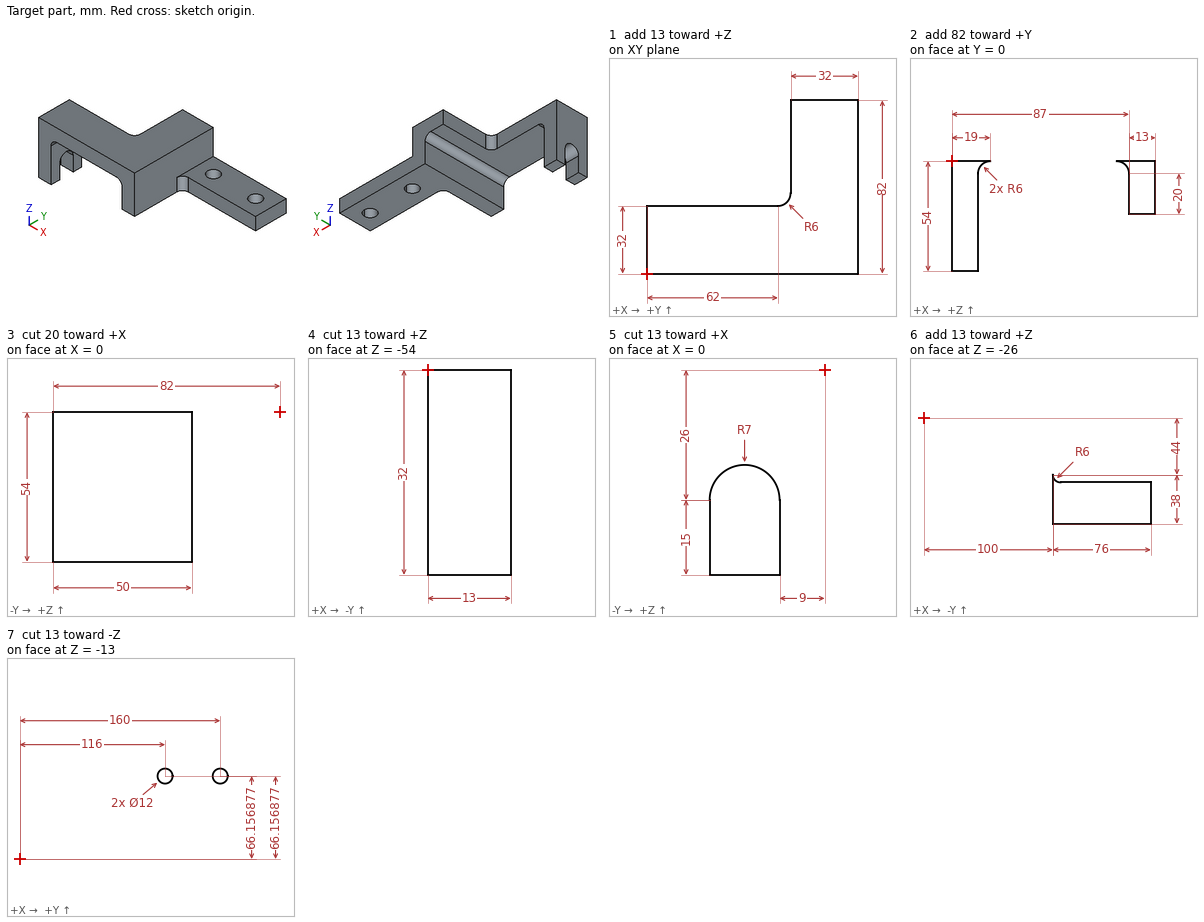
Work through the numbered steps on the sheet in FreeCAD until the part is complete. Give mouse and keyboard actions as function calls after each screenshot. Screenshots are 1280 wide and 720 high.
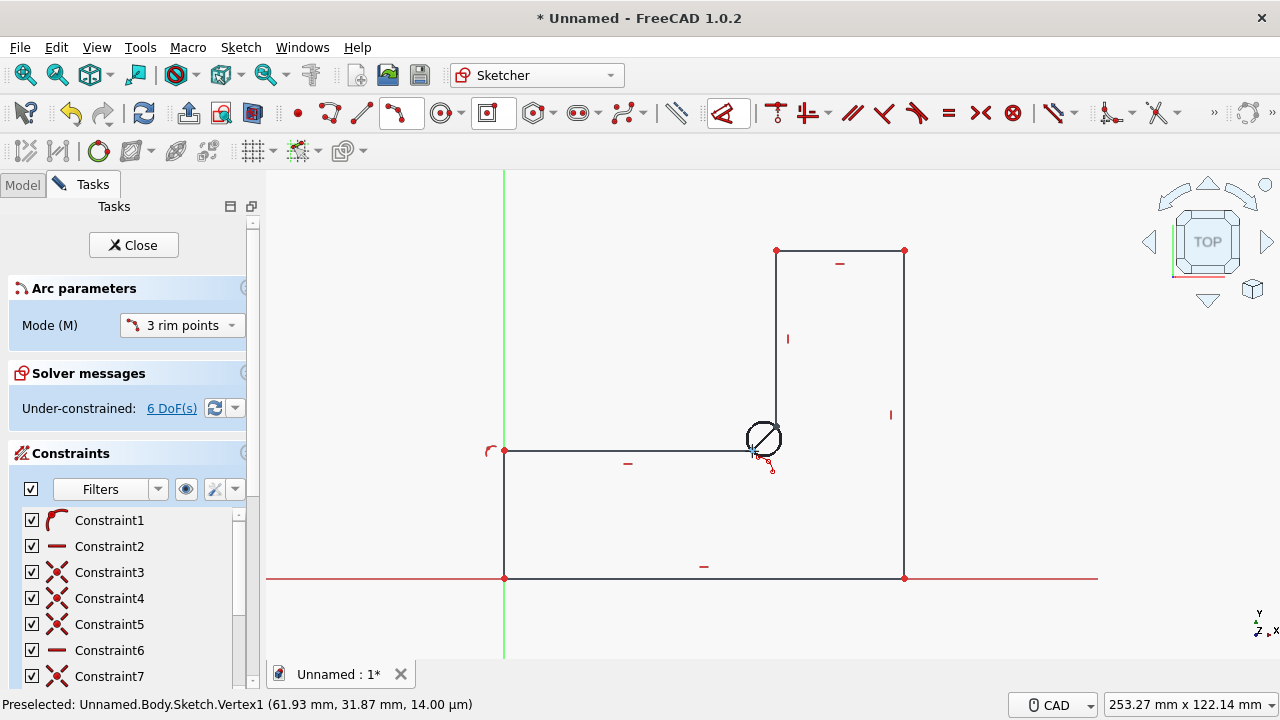
scroll(769, 443, up, 5)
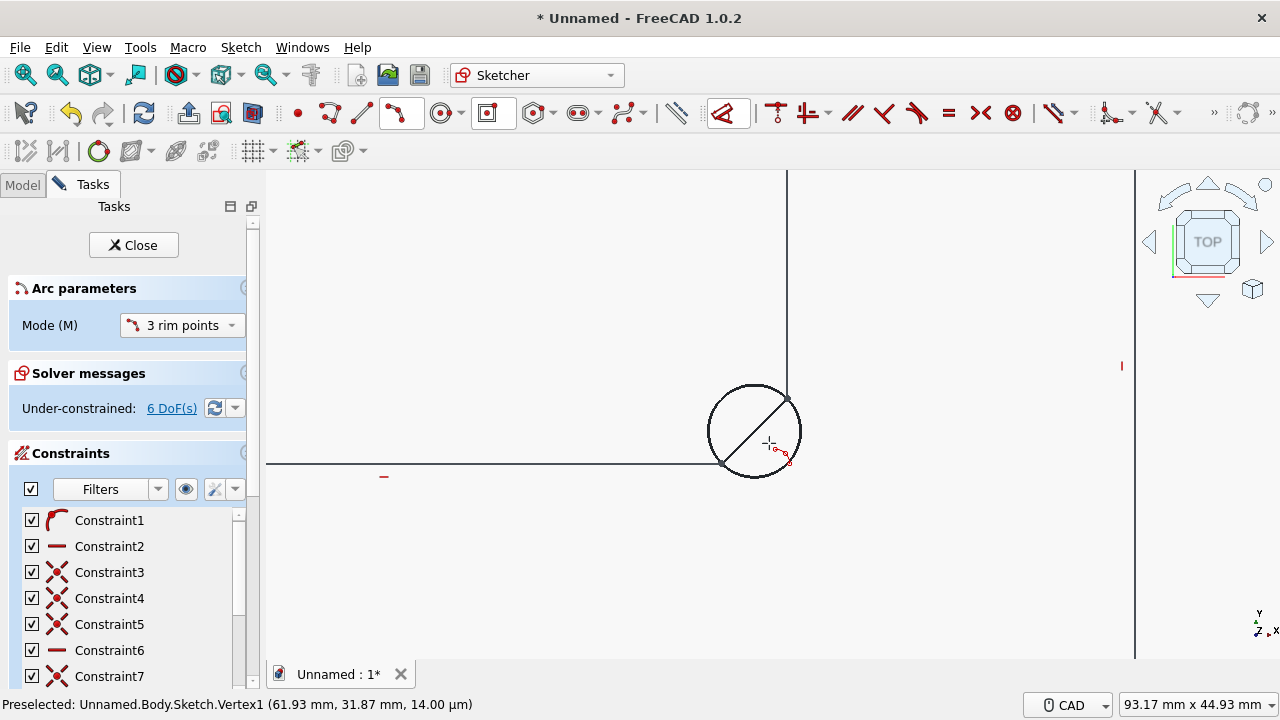
click(769, 443)
key(Escape)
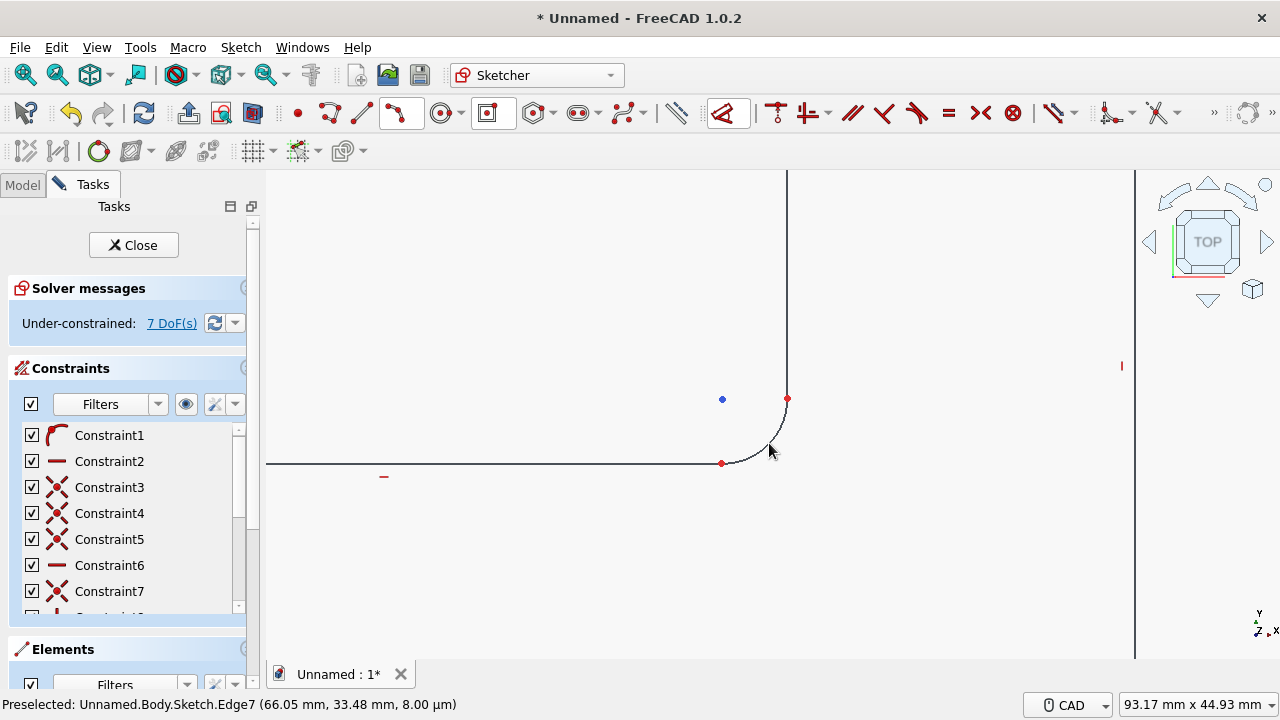
click(520, 464)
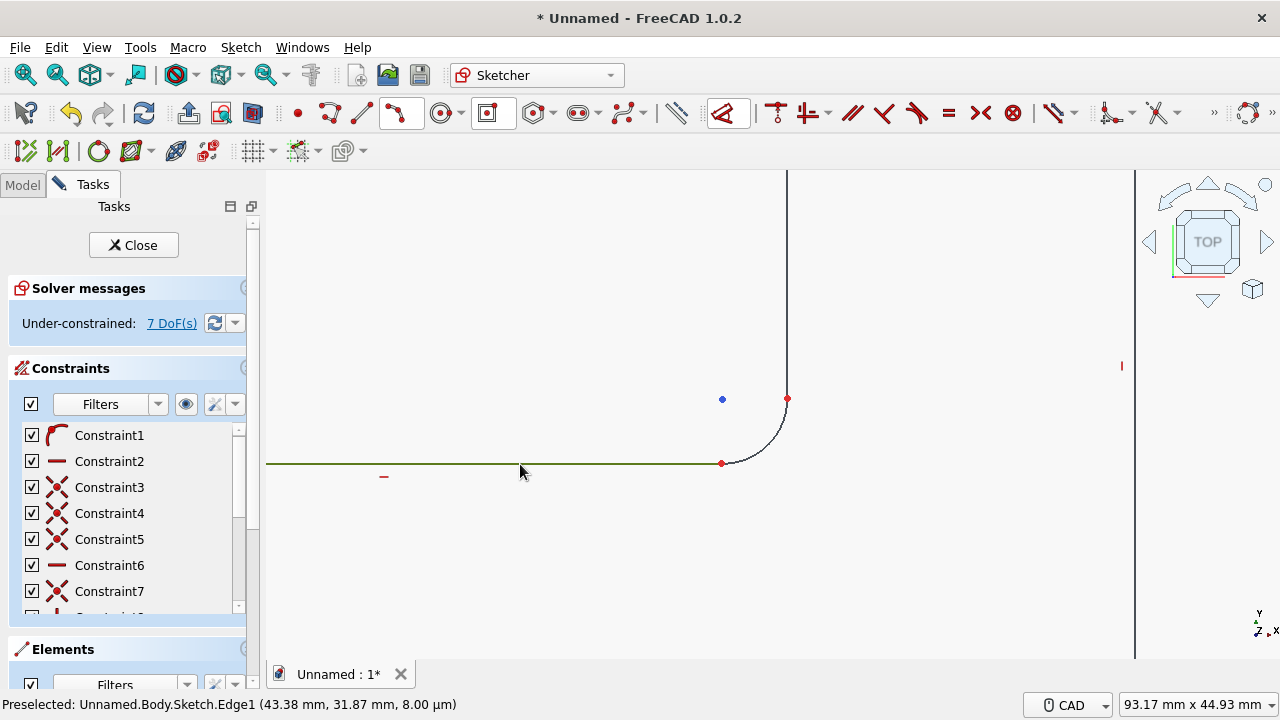
click(752, 457)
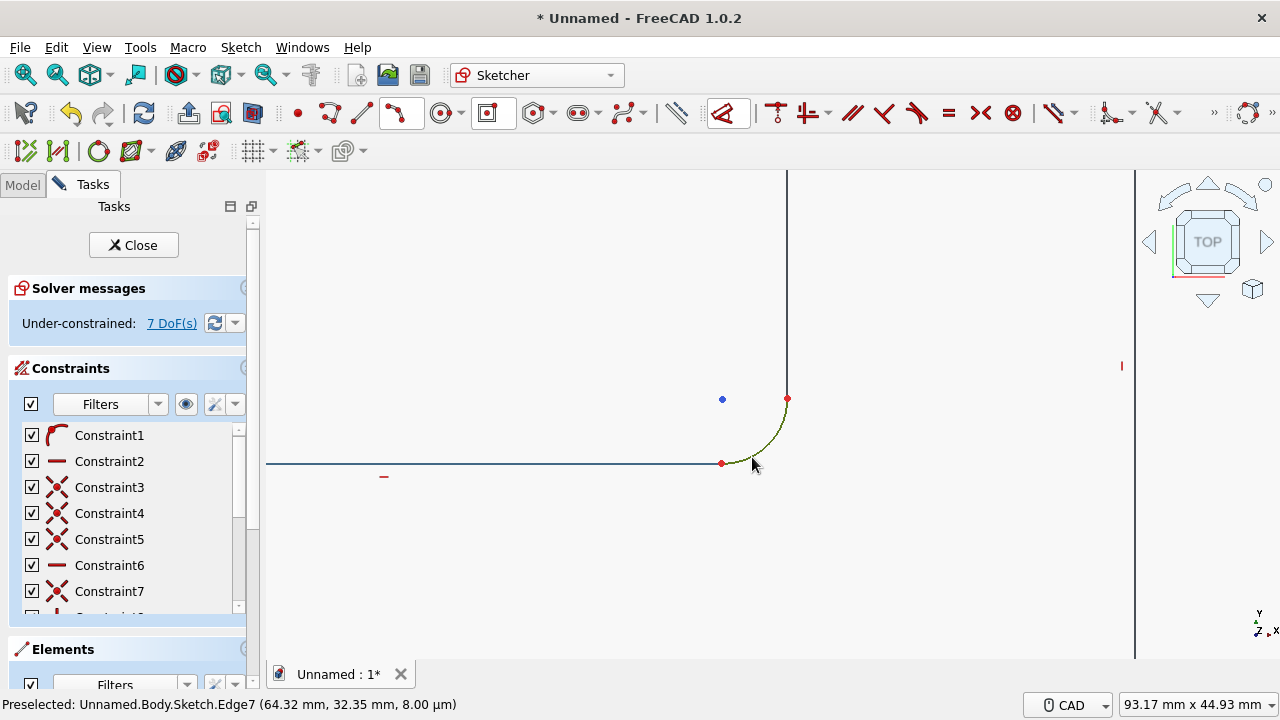
click(918, 114)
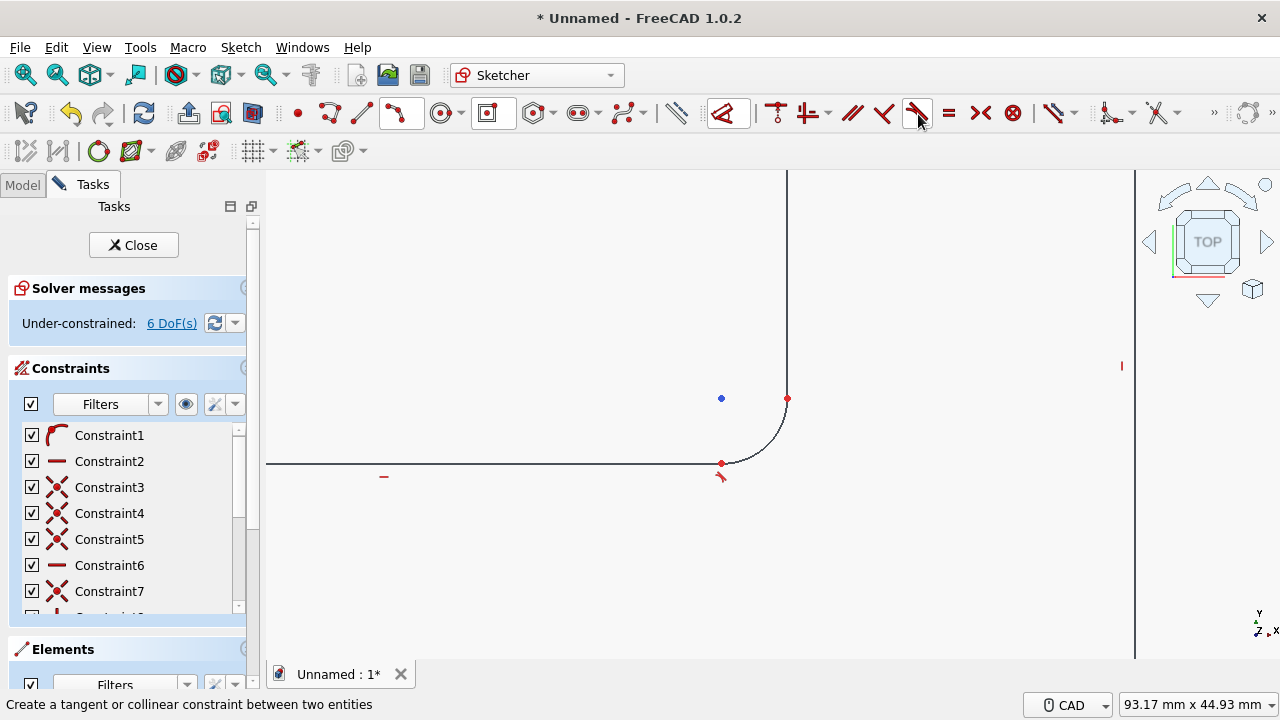
click(787, 255)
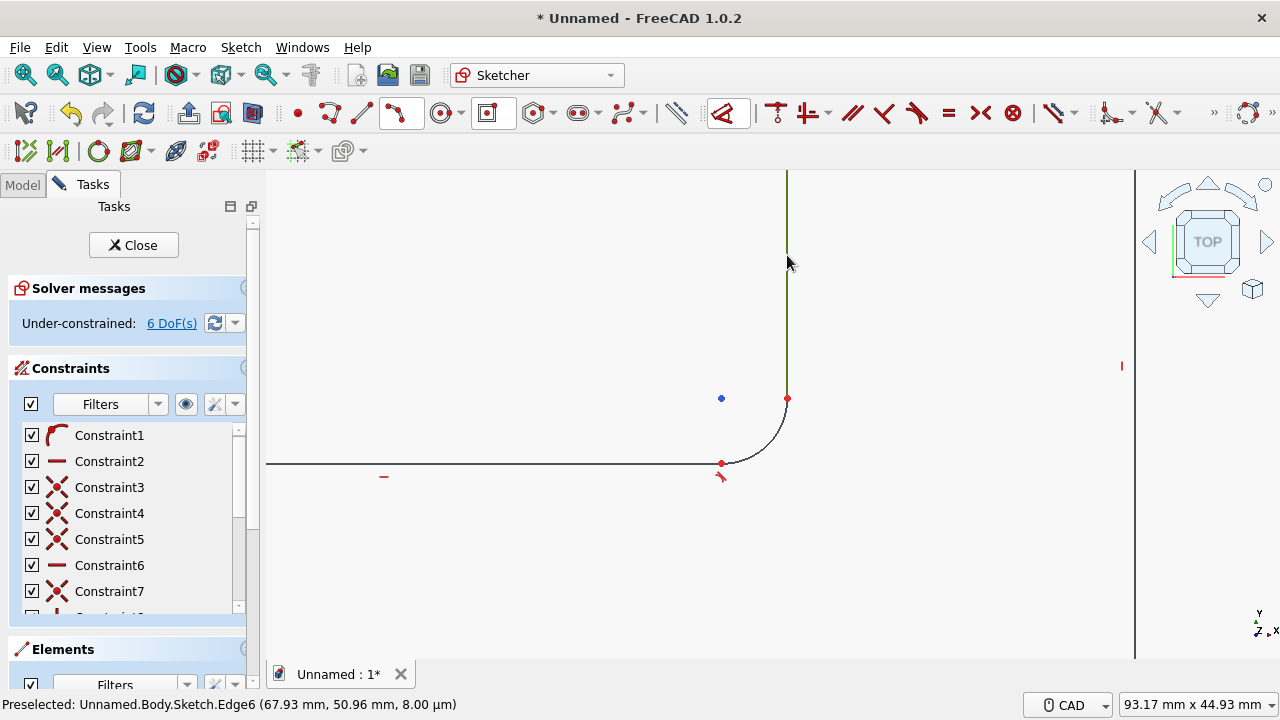
click(752, 457)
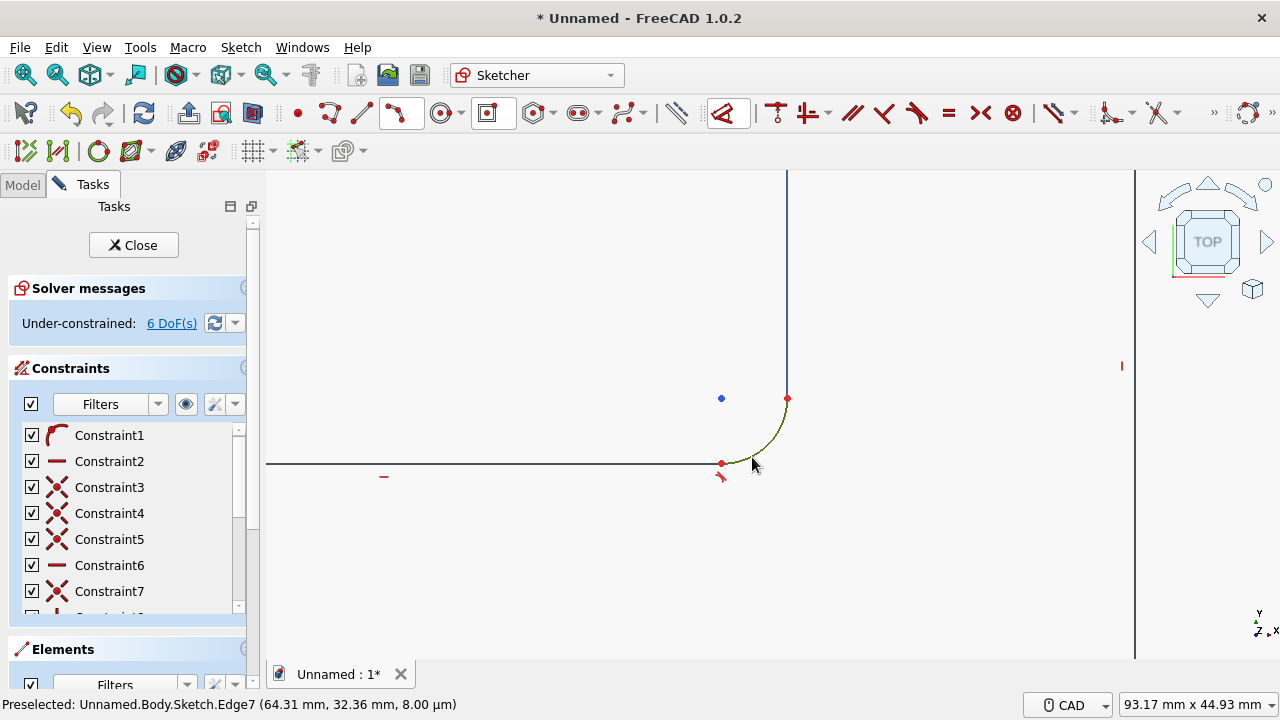
click(918, 114)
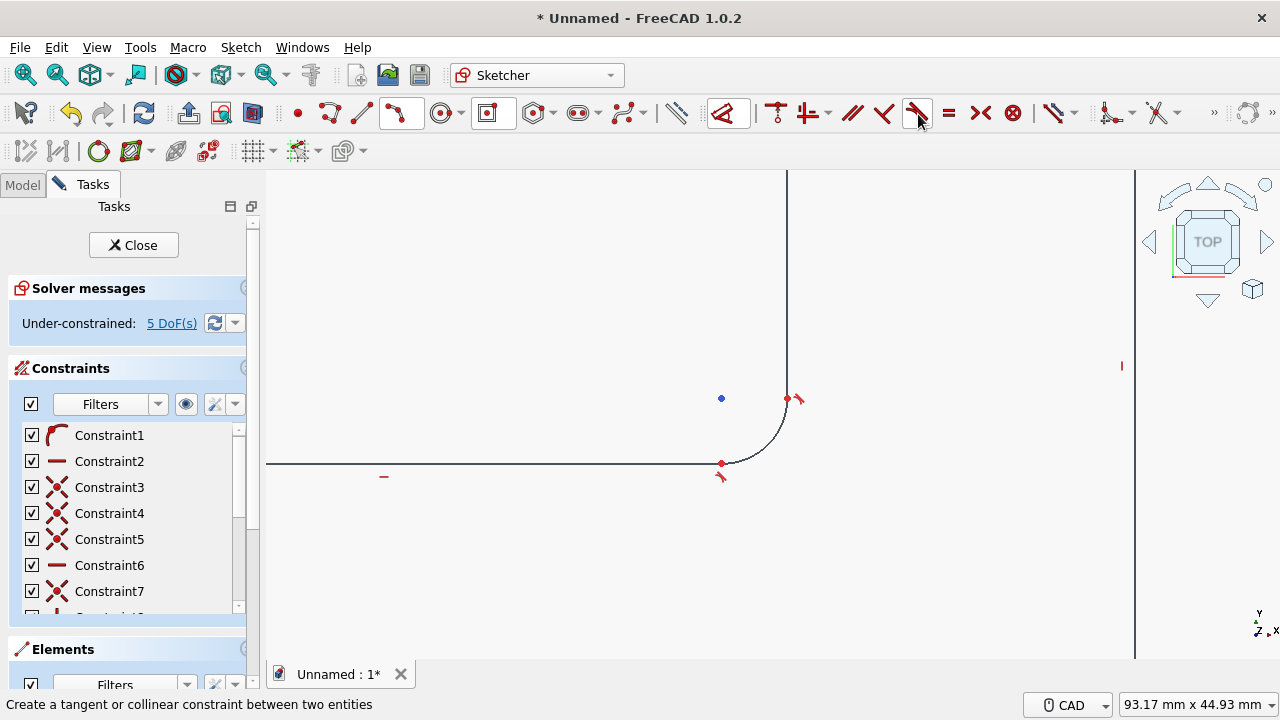
click(722, 114)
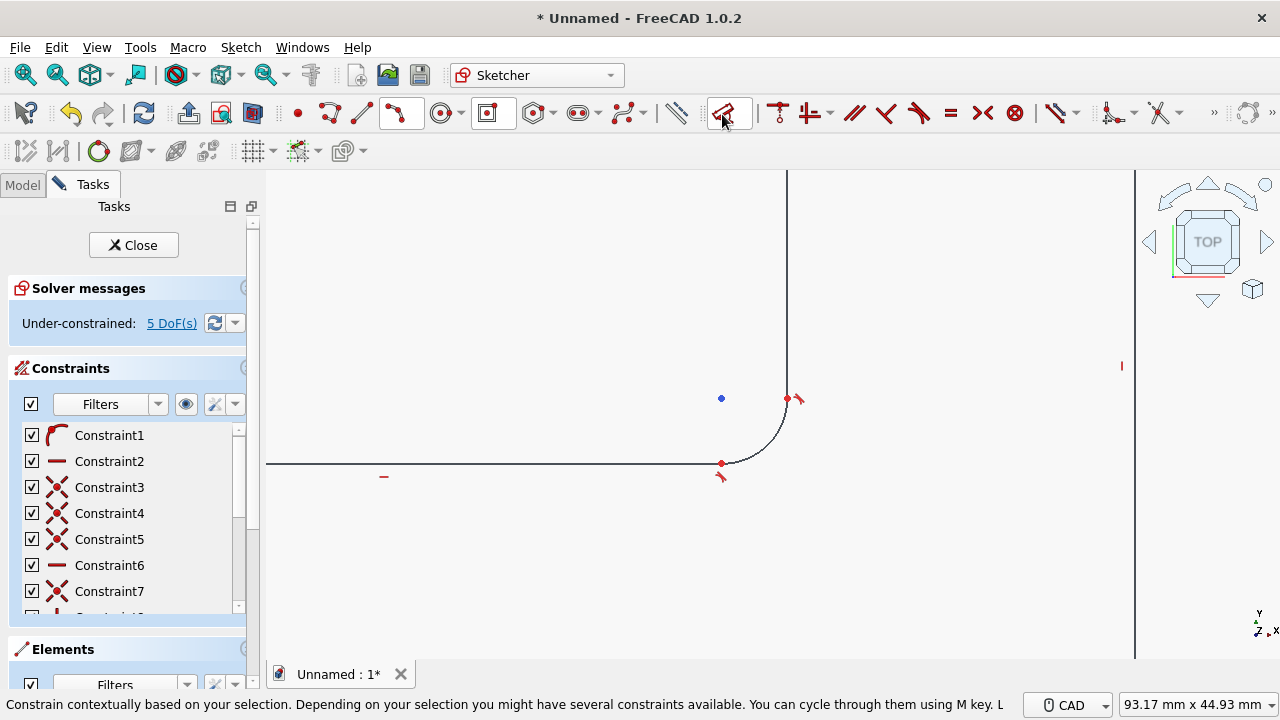
click(752, 457)
click(767, 485)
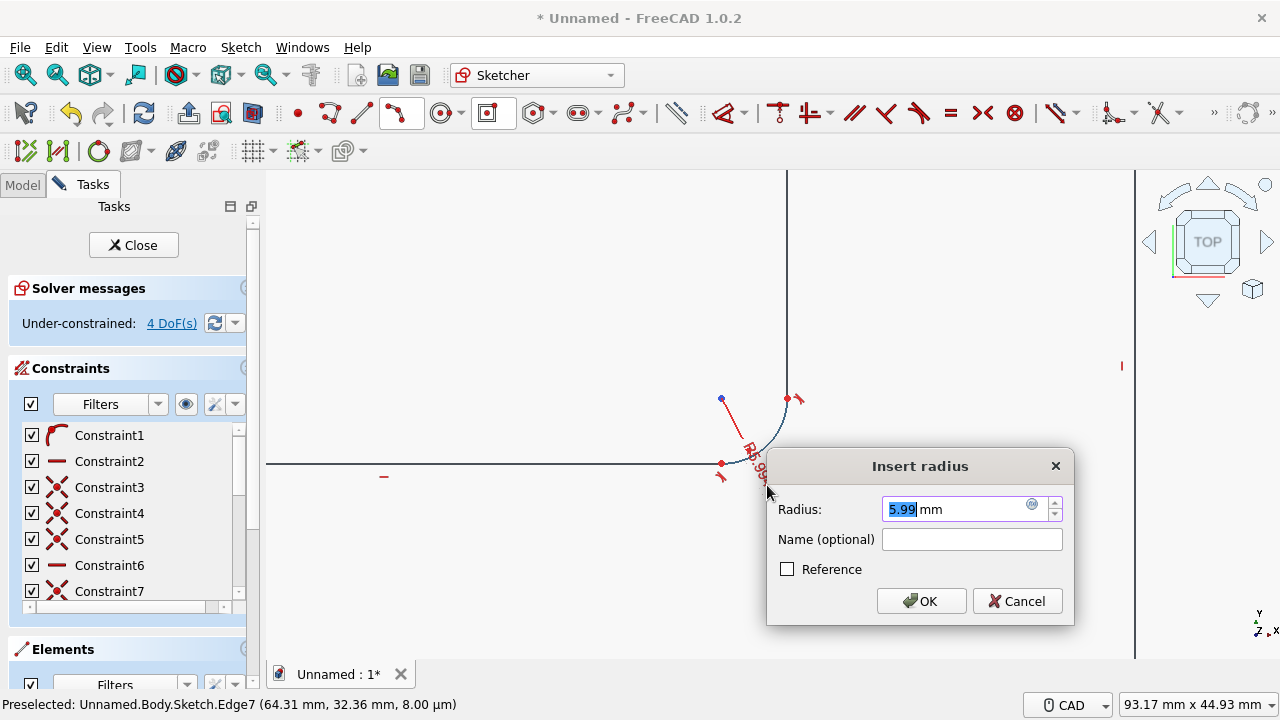
text(6)
key(Return)